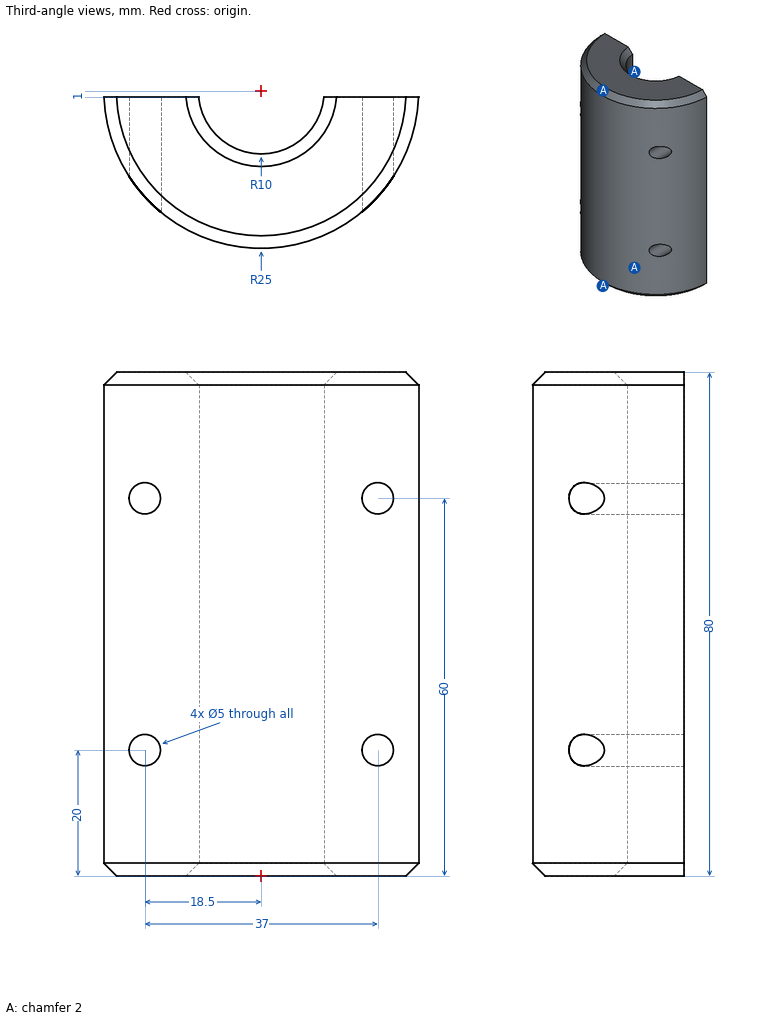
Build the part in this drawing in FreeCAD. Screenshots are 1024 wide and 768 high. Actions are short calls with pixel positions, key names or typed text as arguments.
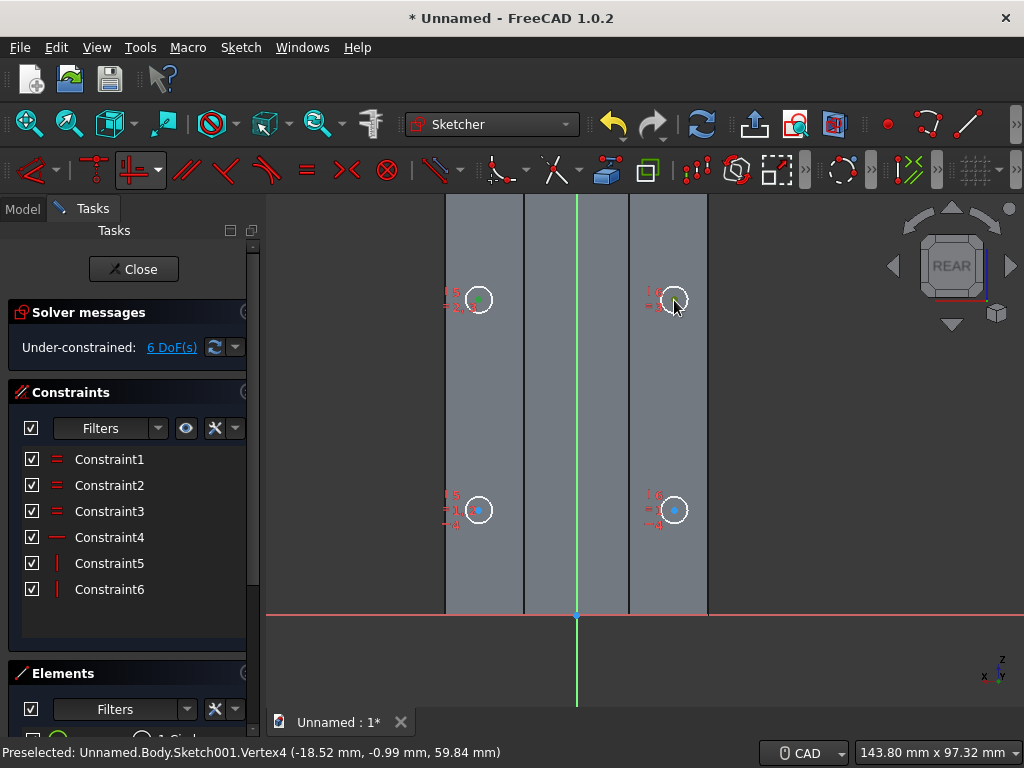
click(160, 170)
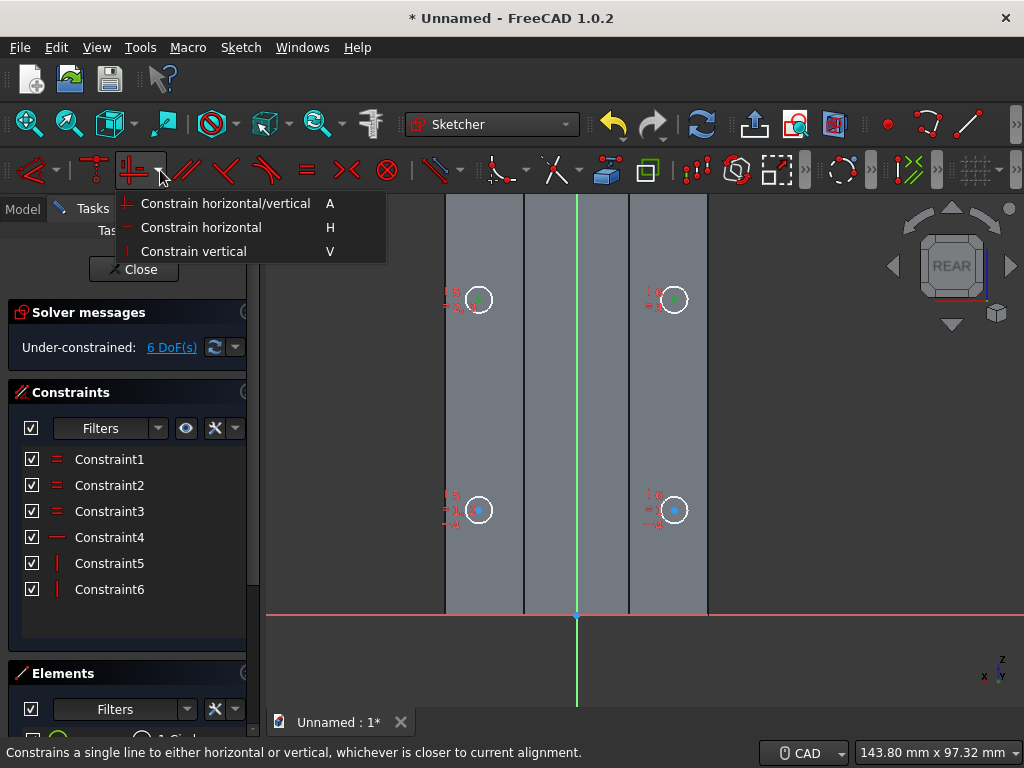
click(251, 227)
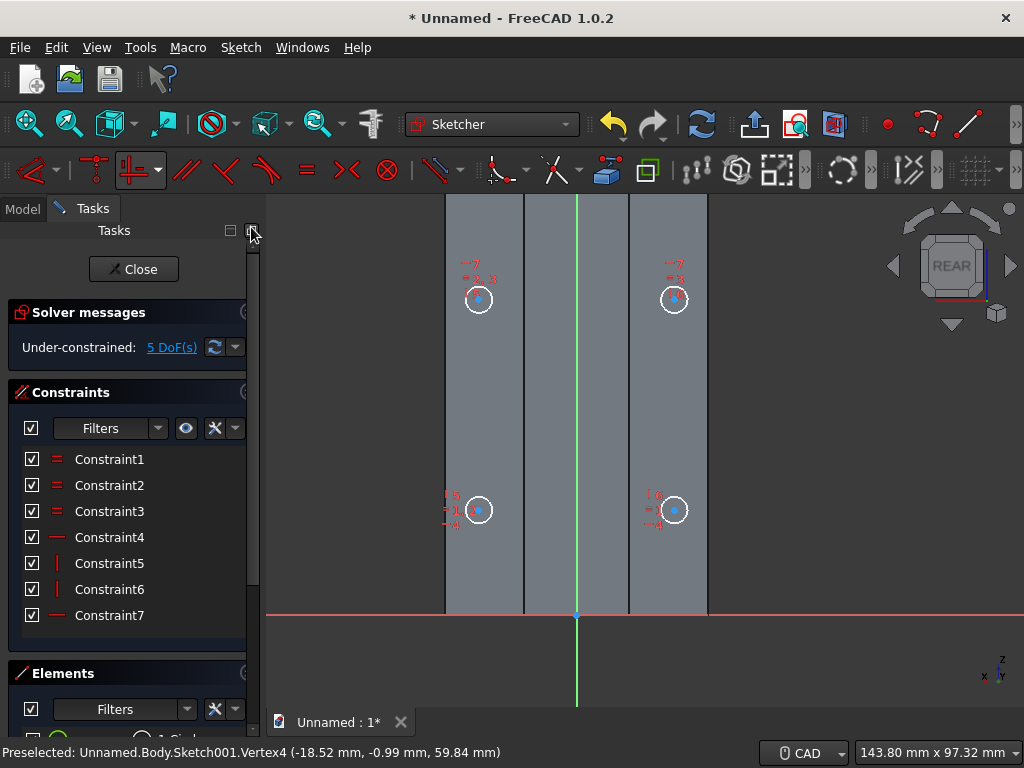
click(32, 170)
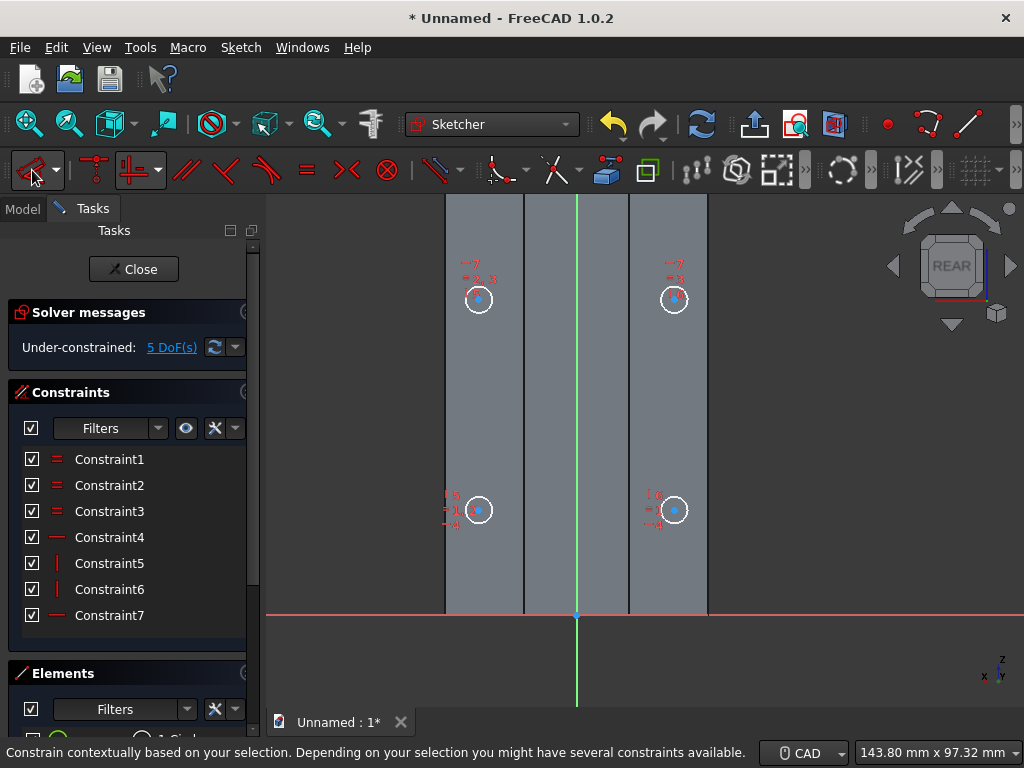
scroll(684, 501, up, 3)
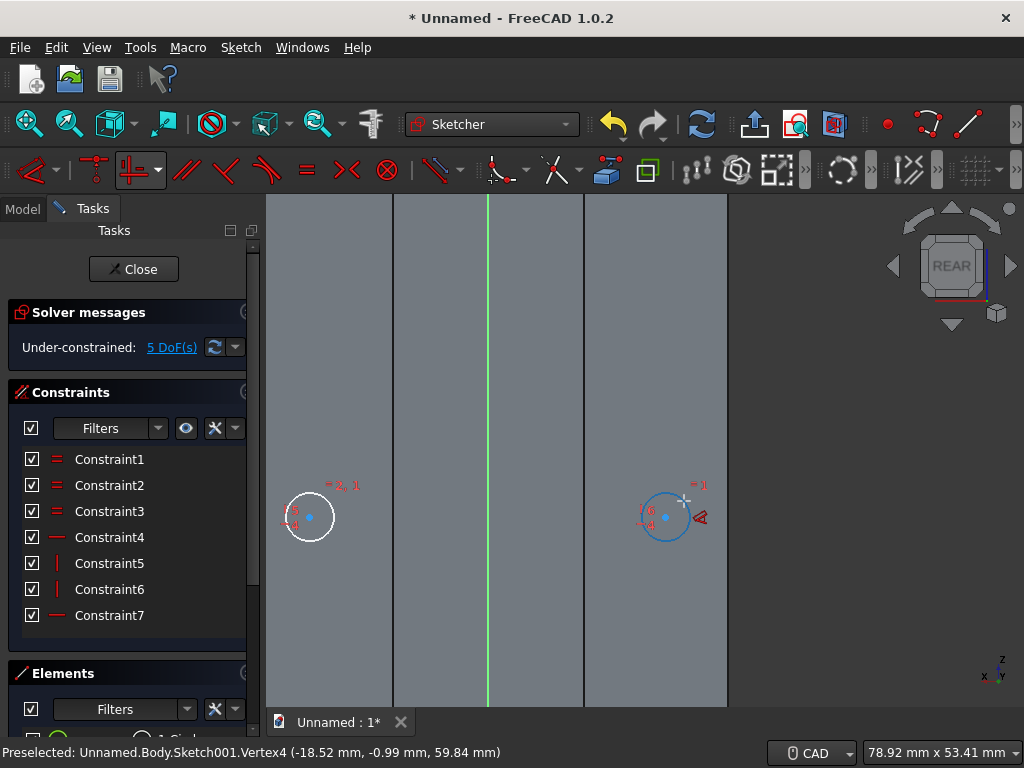
click(683, 500)
click(706, 477)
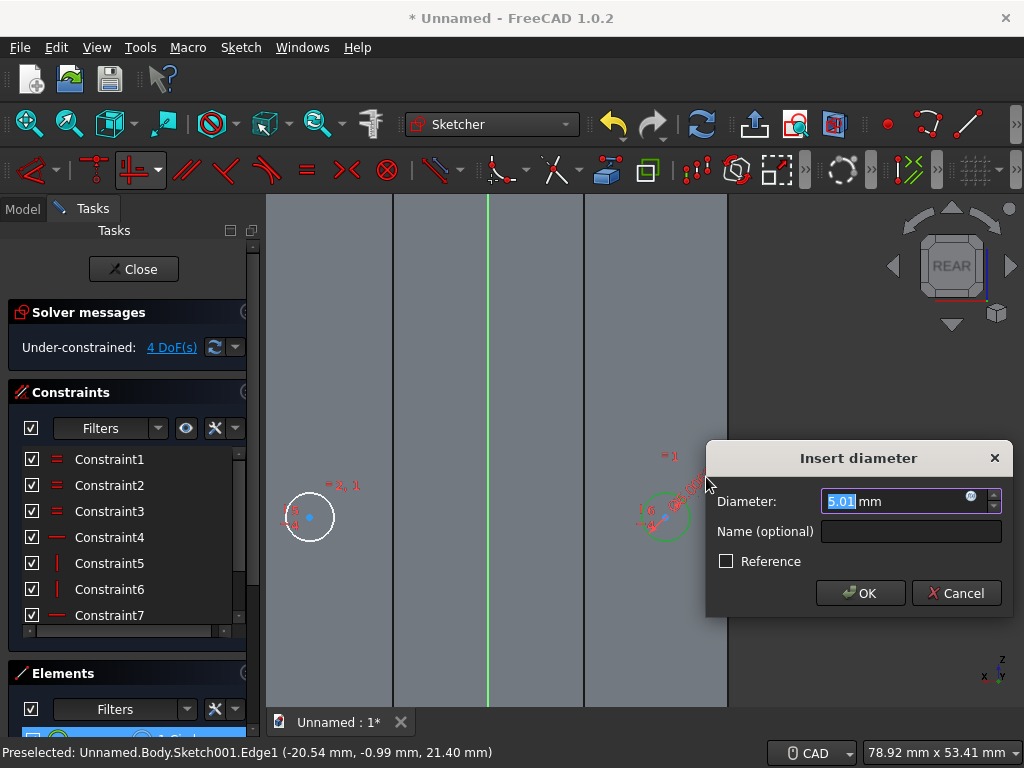
text(5)
key(Return)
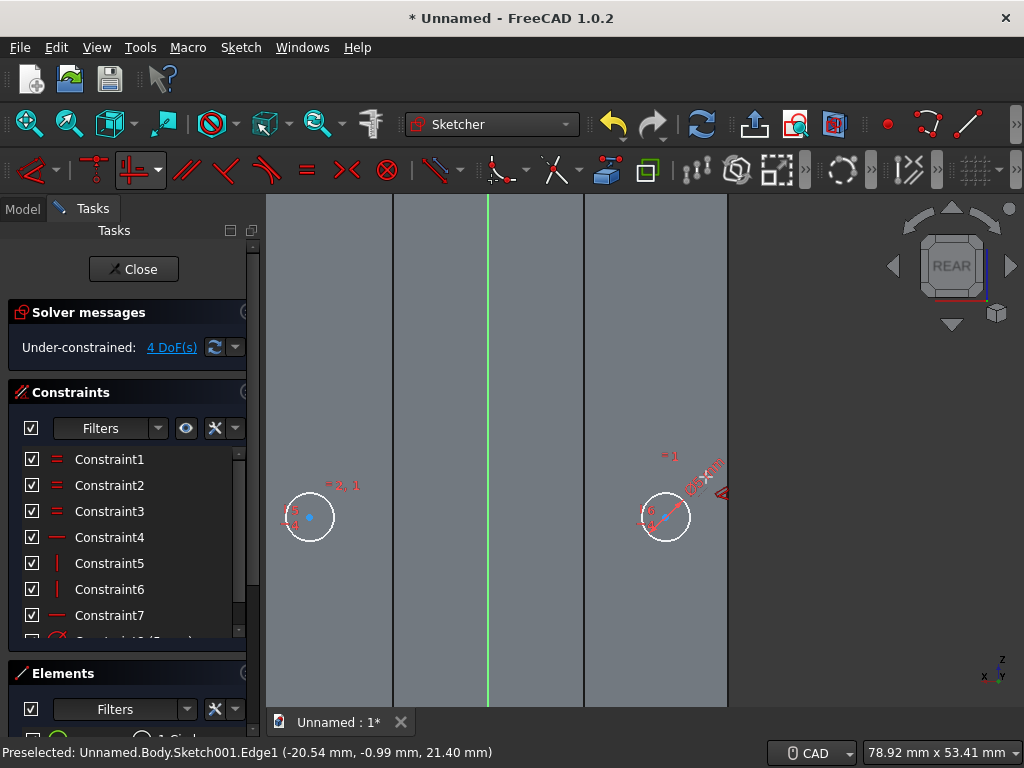
click(666, 517)
click(700, 598)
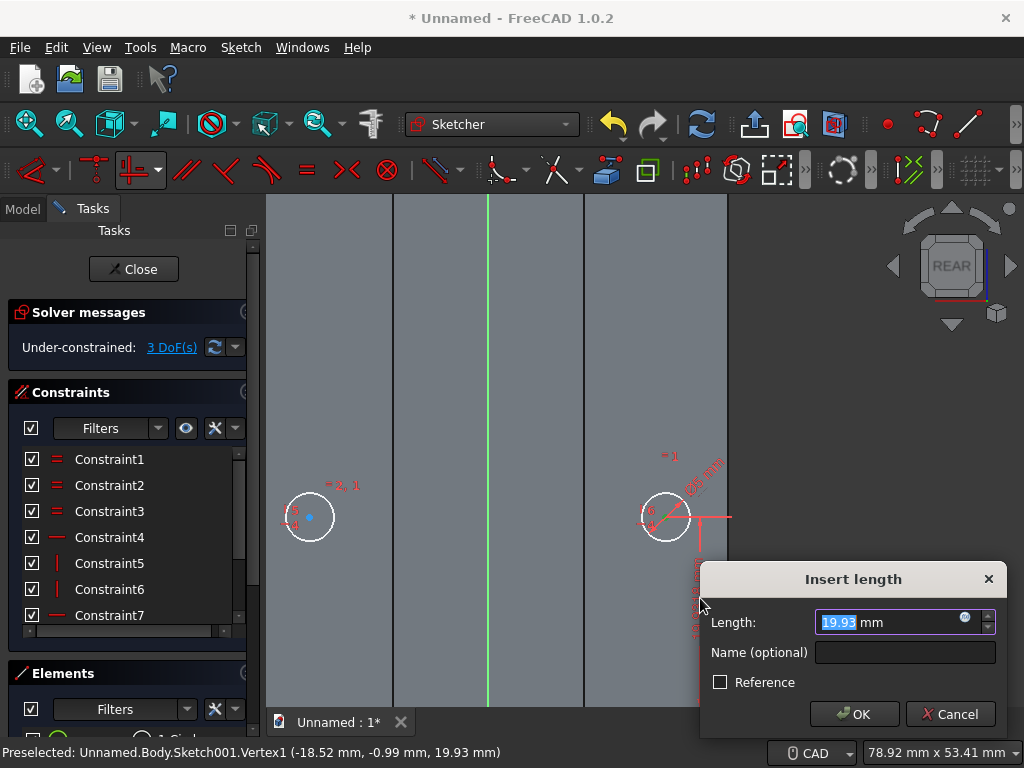
text(20)
key(Return)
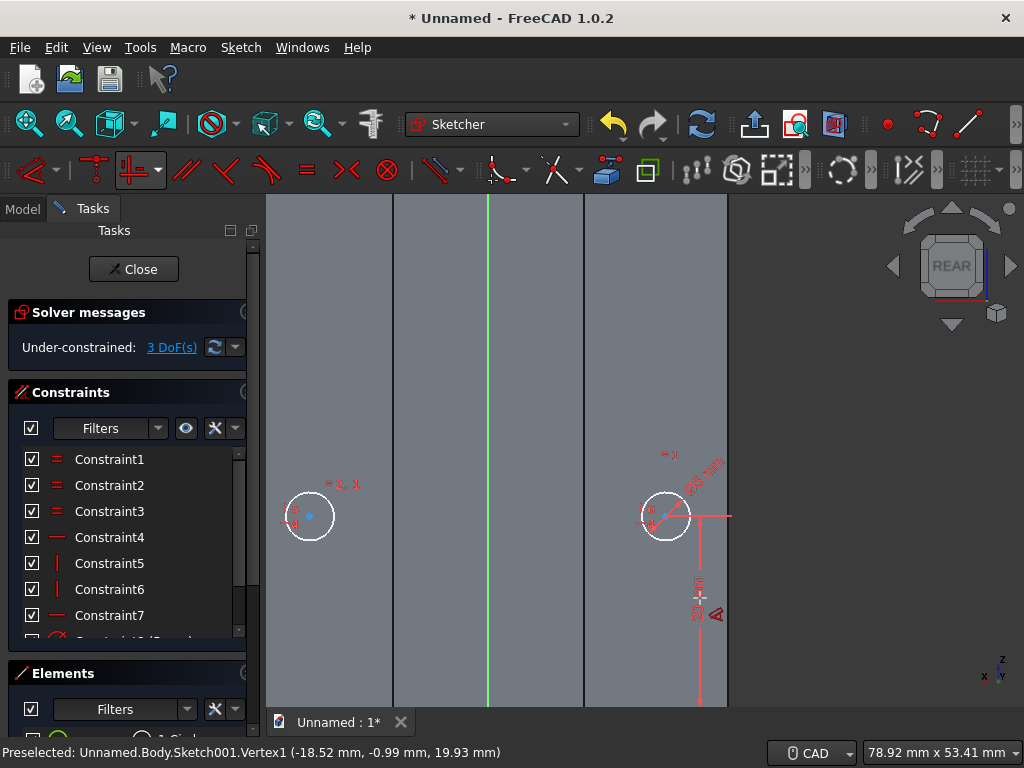
scroll(684, 502, down, 3)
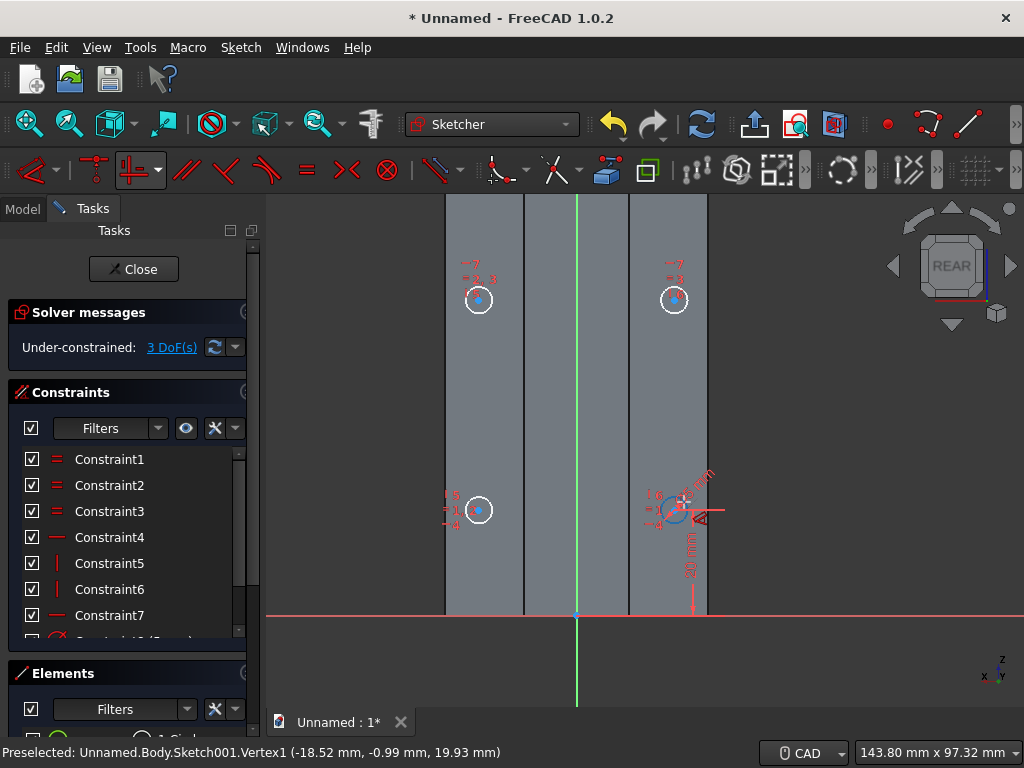
click(479, 300)
click(445, 458)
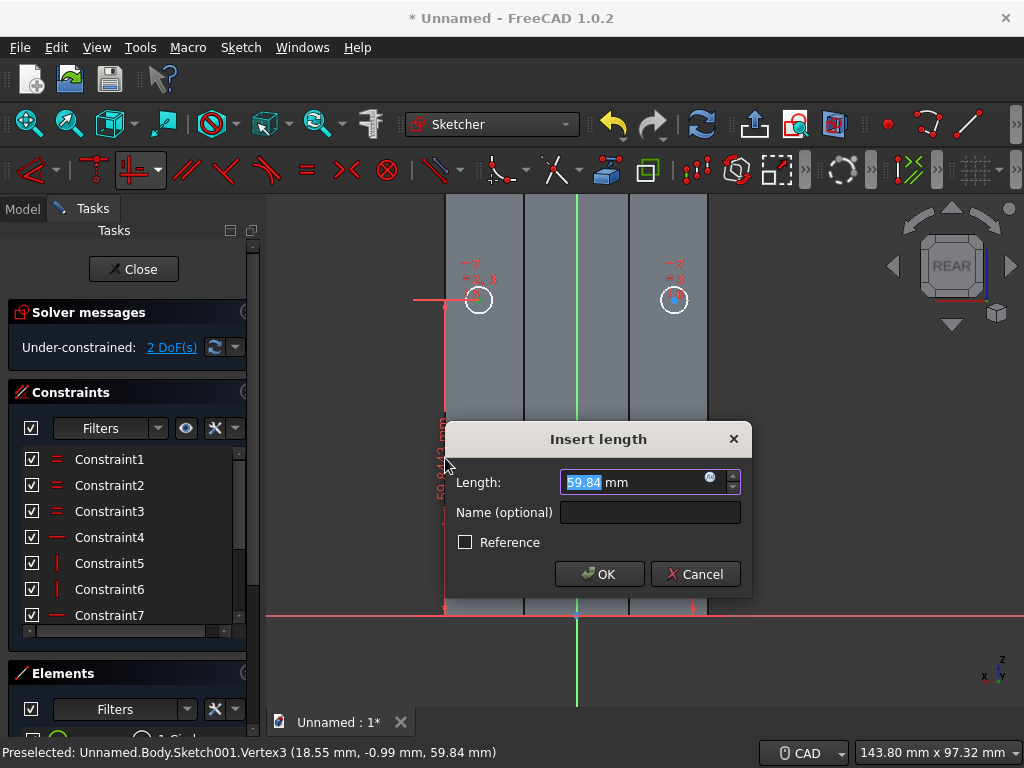
text(60)
key(Return)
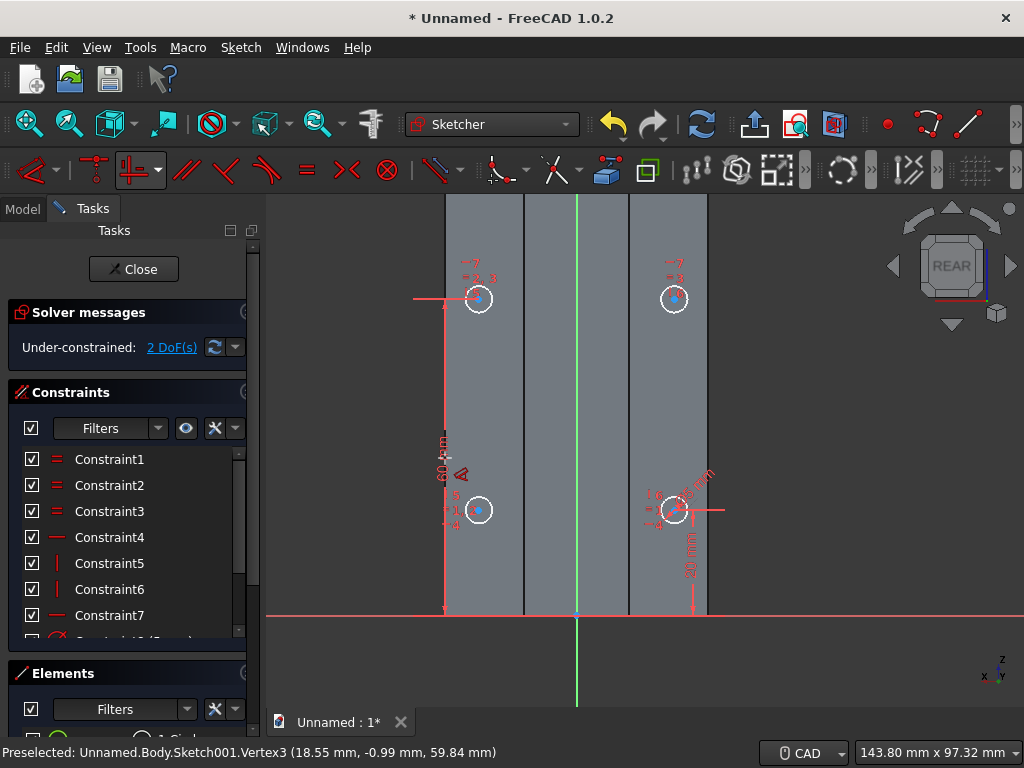
click(674, 510)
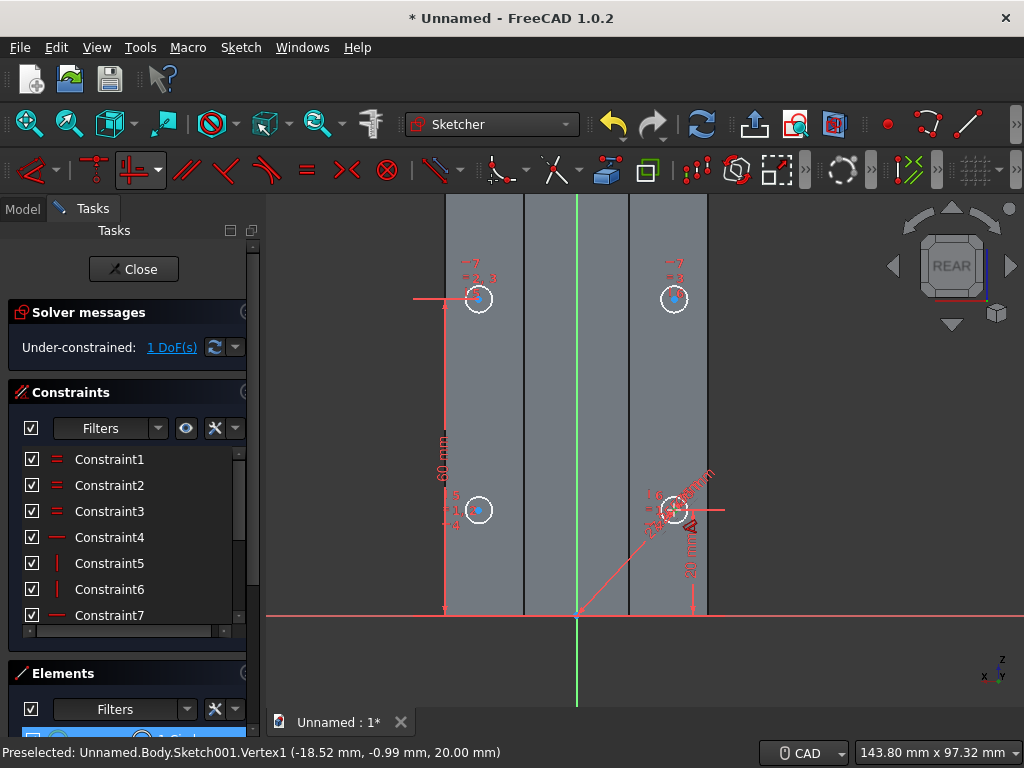
click(479, 510)
click(532, 544)